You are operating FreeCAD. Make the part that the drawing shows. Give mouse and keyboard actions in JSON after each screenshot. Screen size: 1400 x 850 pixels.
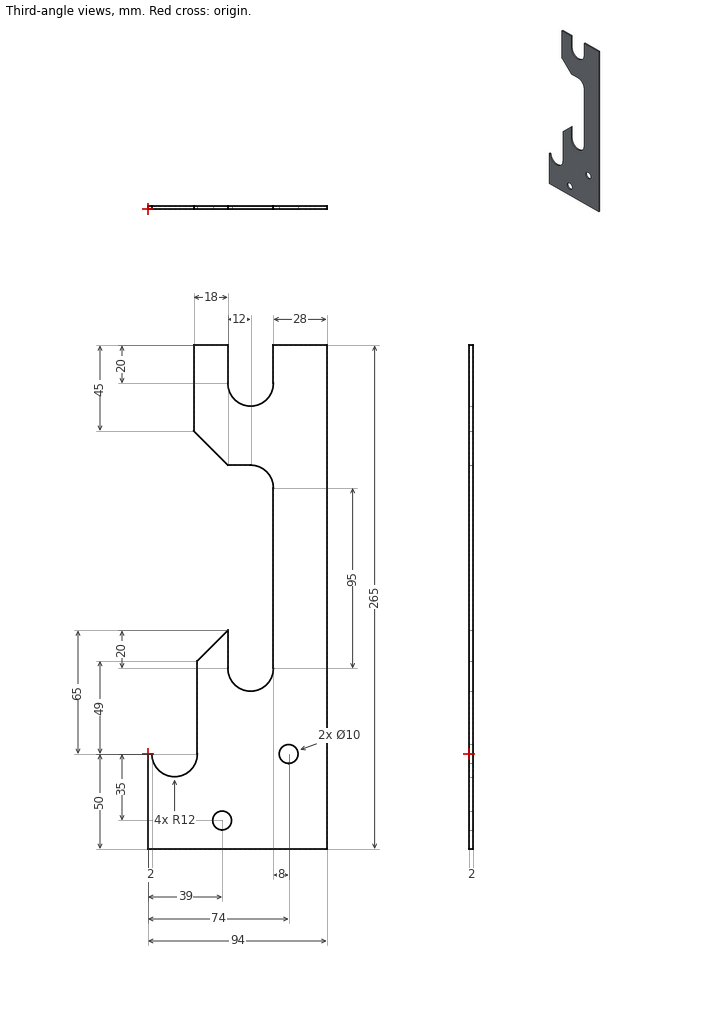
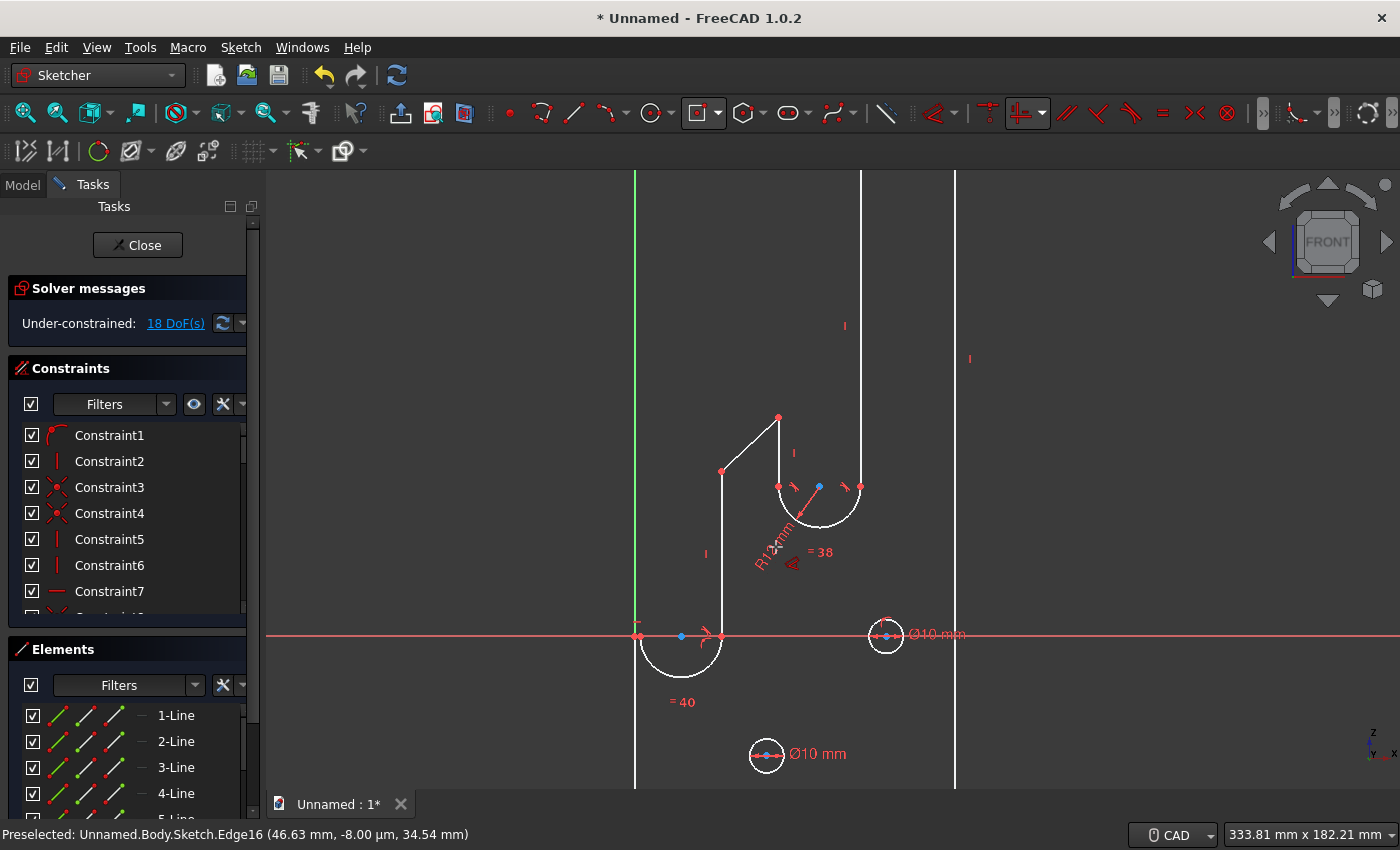
{"action": "scroll", "coordinate": [637, 636], "scroll_direction": "up", "scroll_amount": 9}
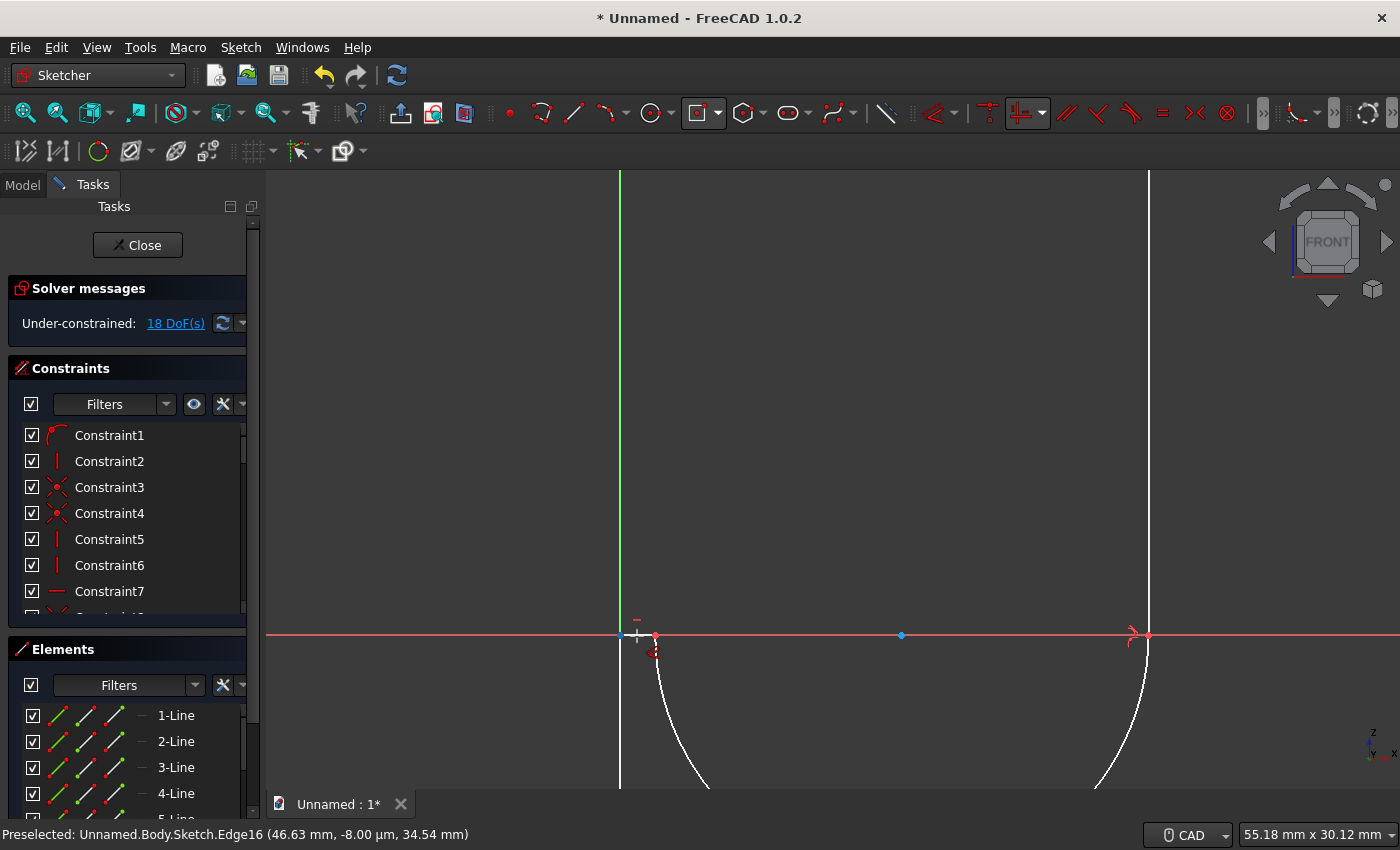
{"action": "left_click", "coordinate": [638, 635]}
{"action": "left_click", "coordinate": [638, 669]}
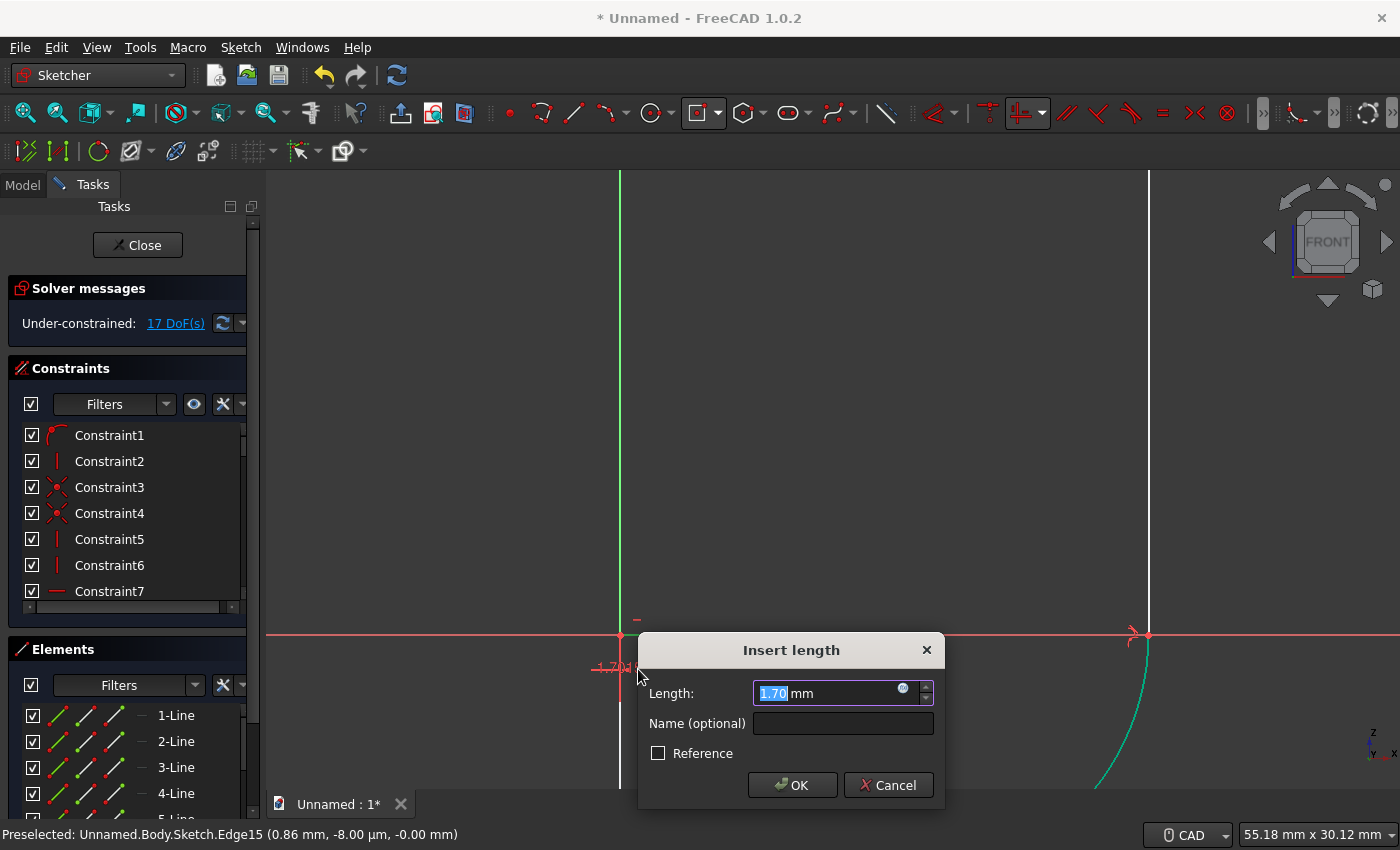
{"action": "type", "text": "2"}
{"action": "key", "text": "Return"}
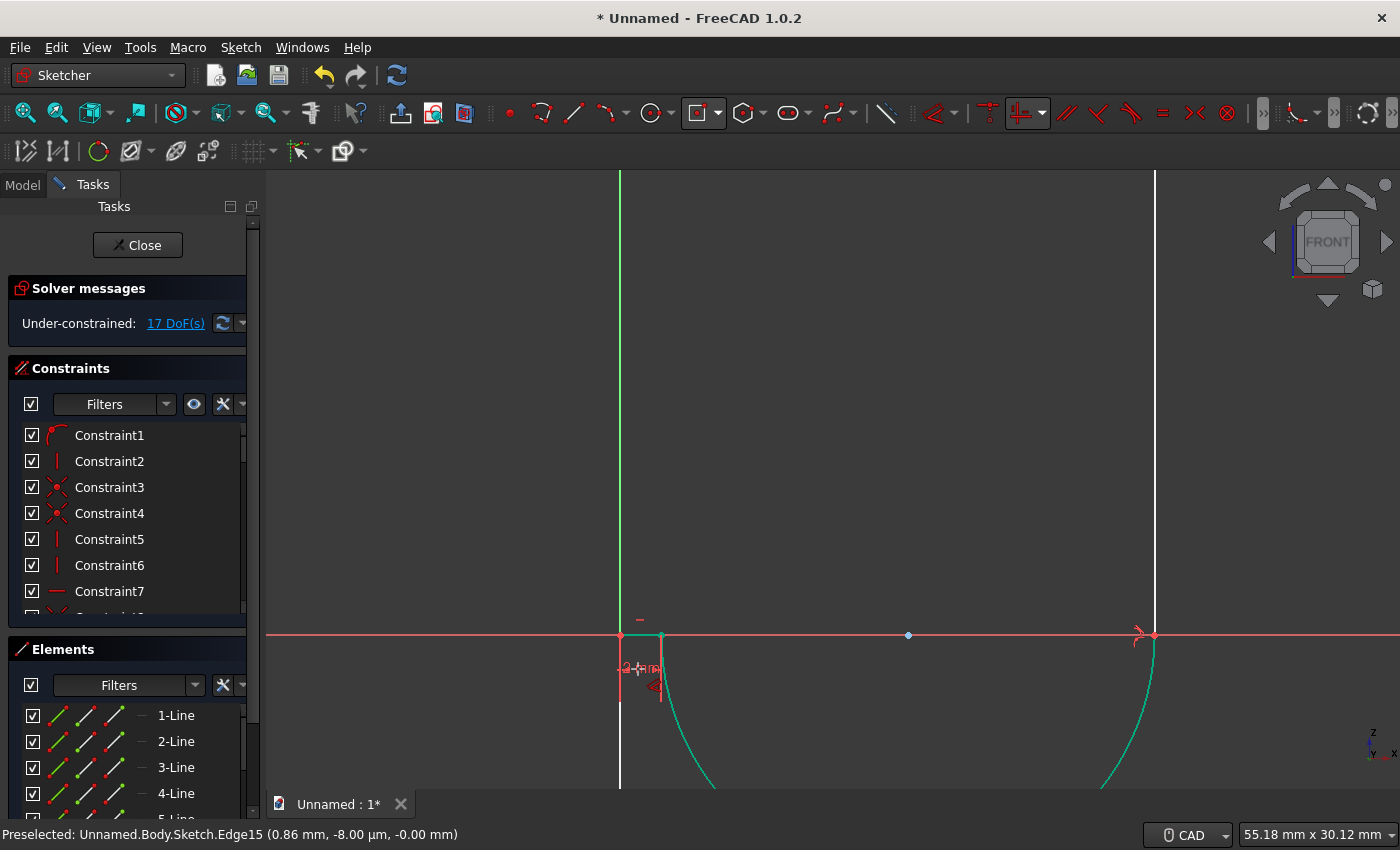
{"action": "scroll", "coordinate": [699, 603], "scroll_direction": "down", "scroll_amount": 13}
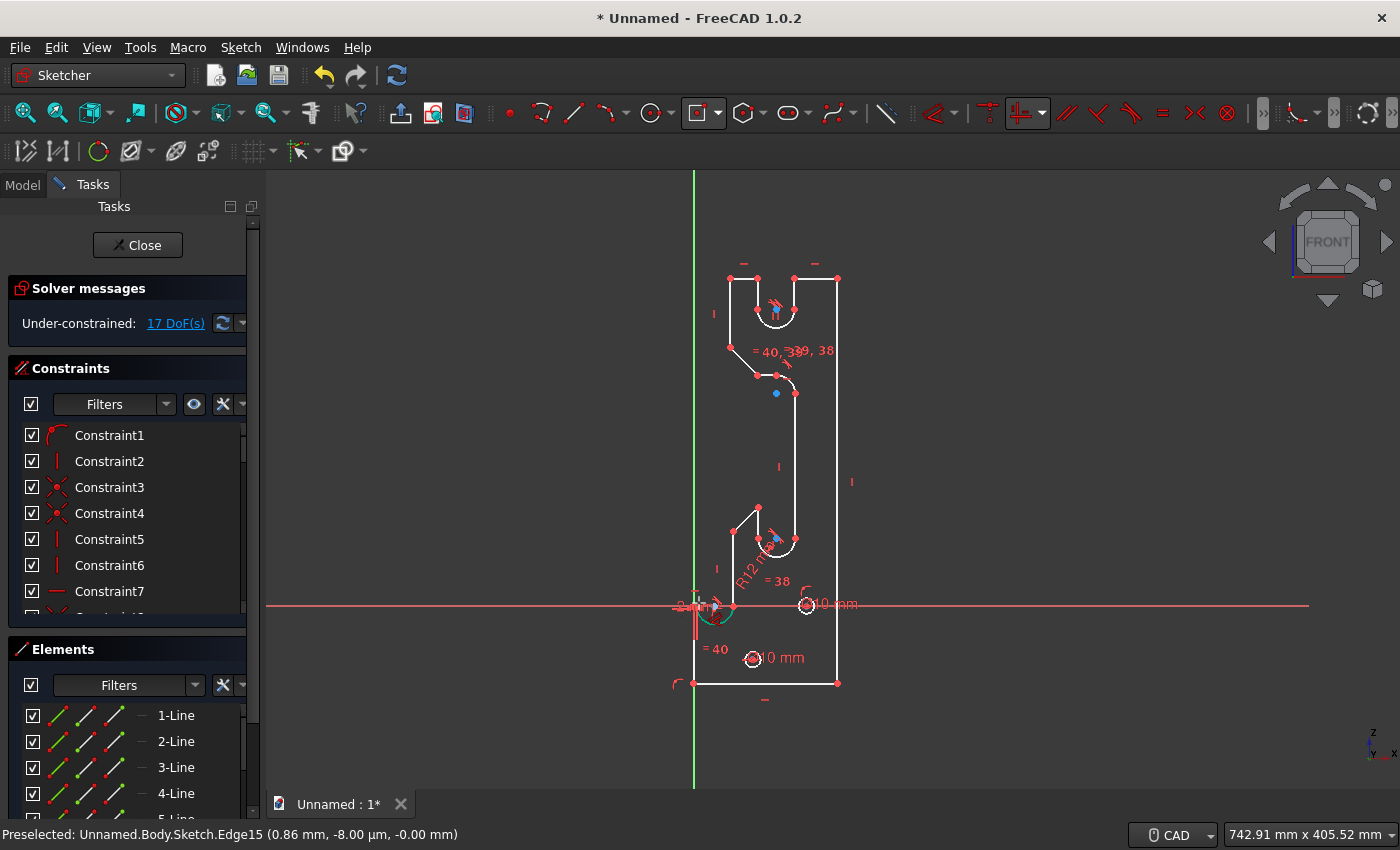
{"action": "left_click", "coordinate": [733, 584]}
{"action": "left_click", "coordinate": [767, 586]}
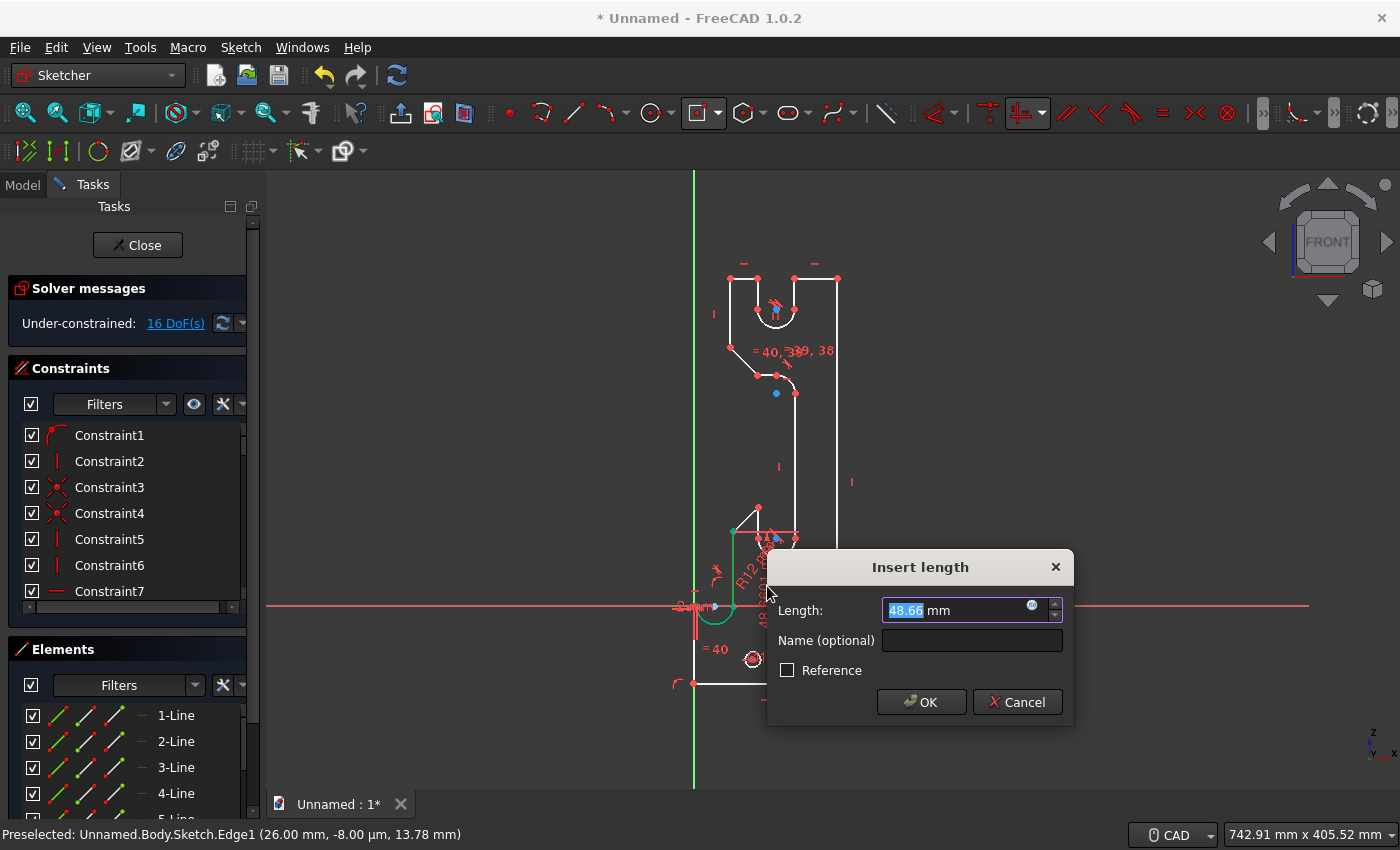
{"action": "type", "text": "49"}
{"action": "key", "text": "Return"}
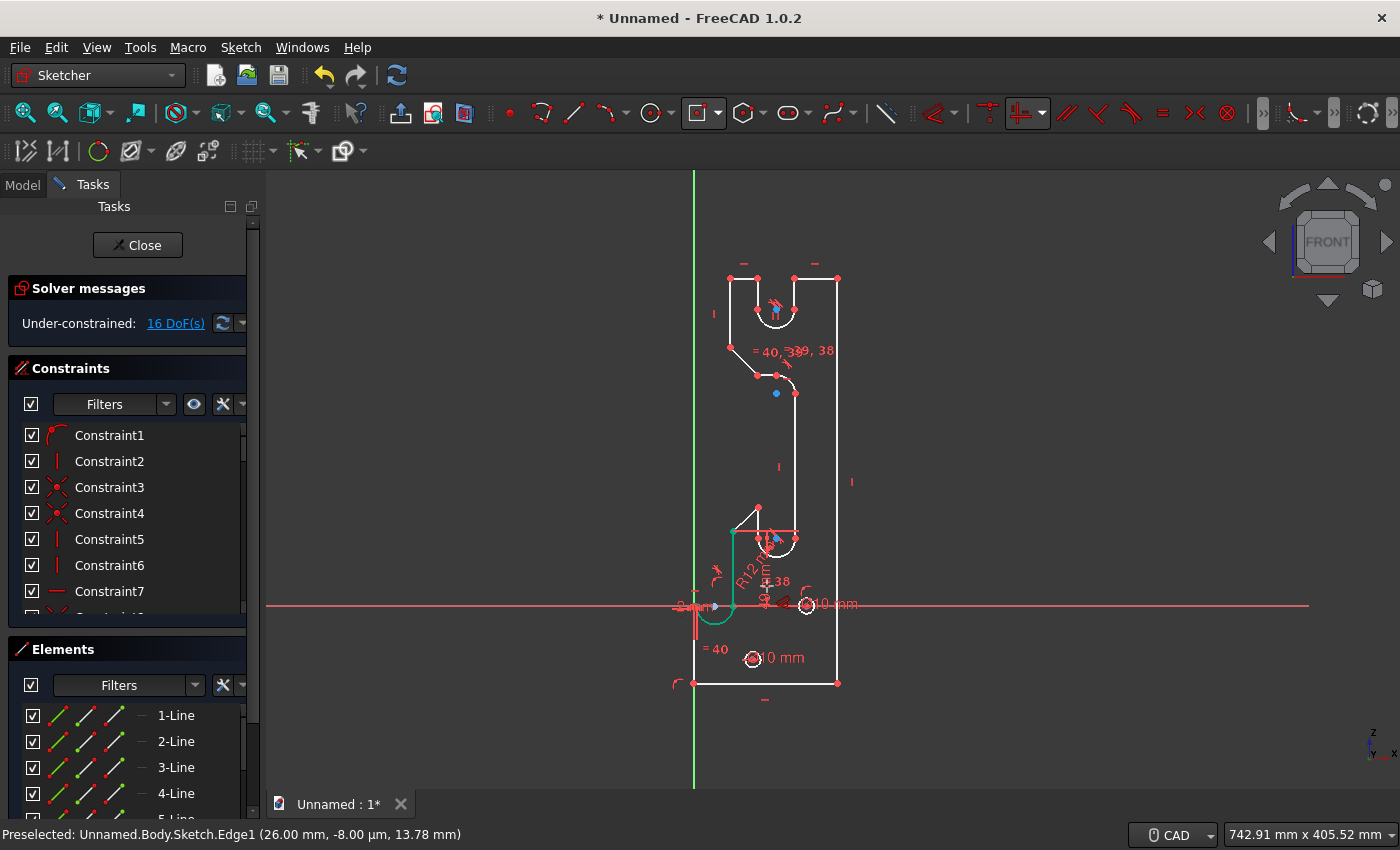
{"action": "scroll", "coordinate": [758, 529], "scroll_direction": "up", "scroll_amount": 2}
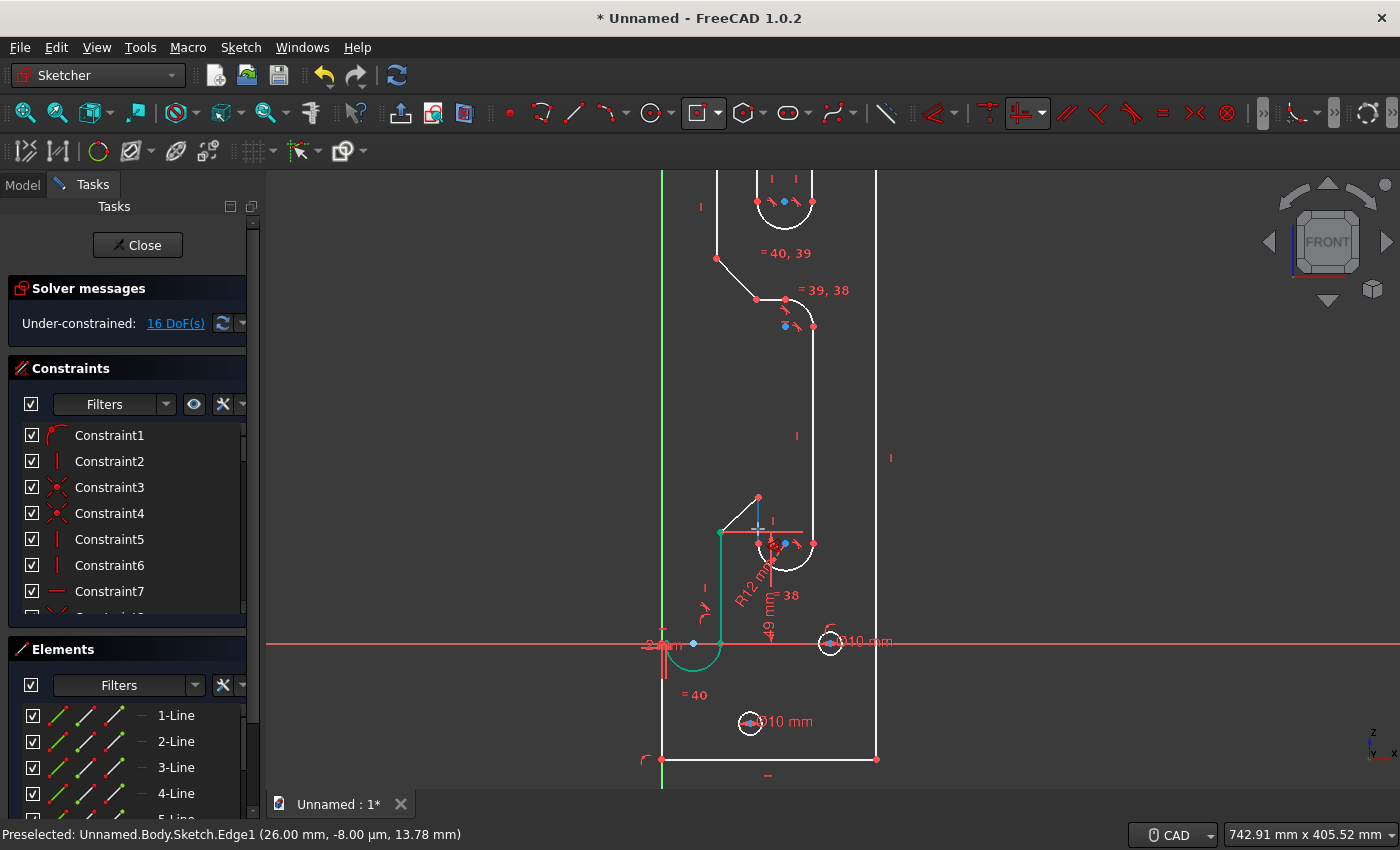
{"action": "left_click", "coordinate": [758, 529]}
{"action": "left_click", "coordinate": [724, 510]}